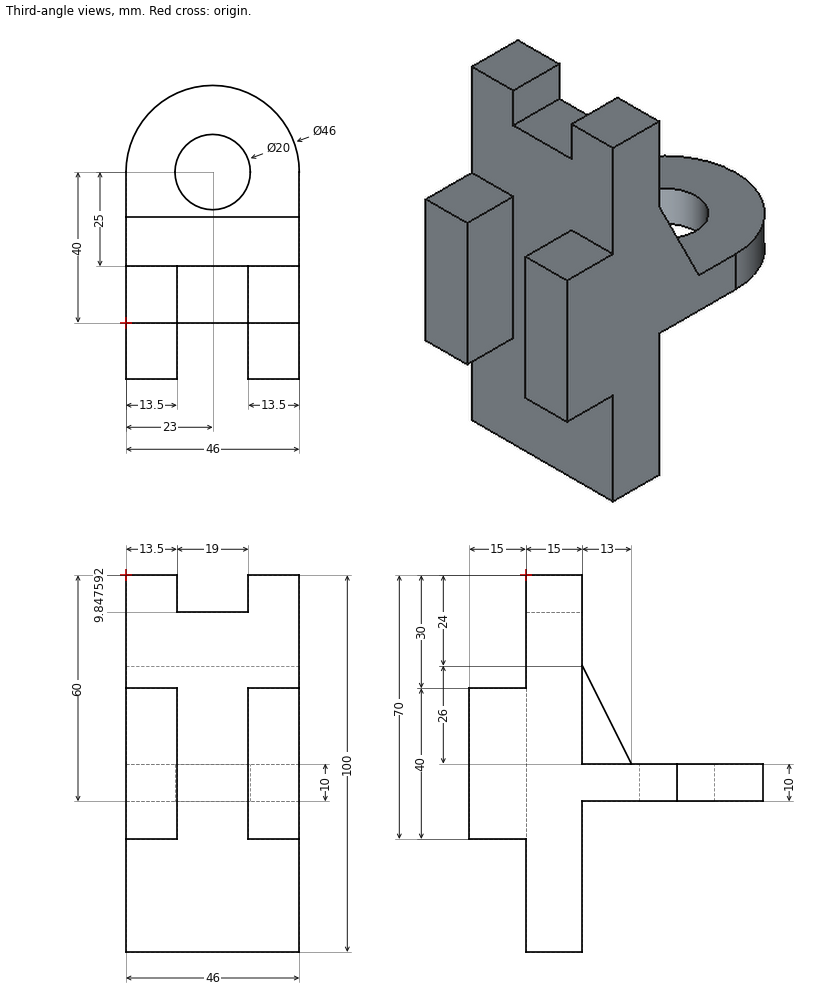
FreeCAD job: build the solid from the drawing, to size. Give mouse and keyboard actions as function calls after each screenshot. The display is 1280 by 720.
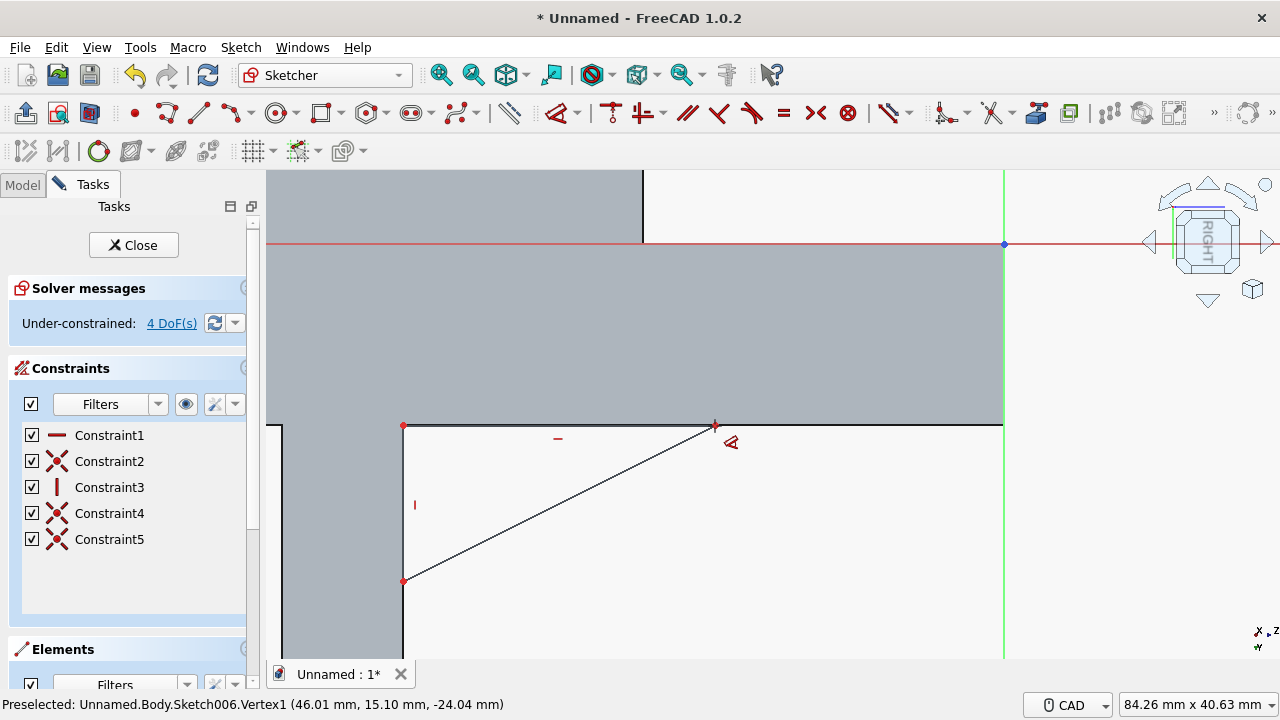
click(621, 426)
click(559, 460)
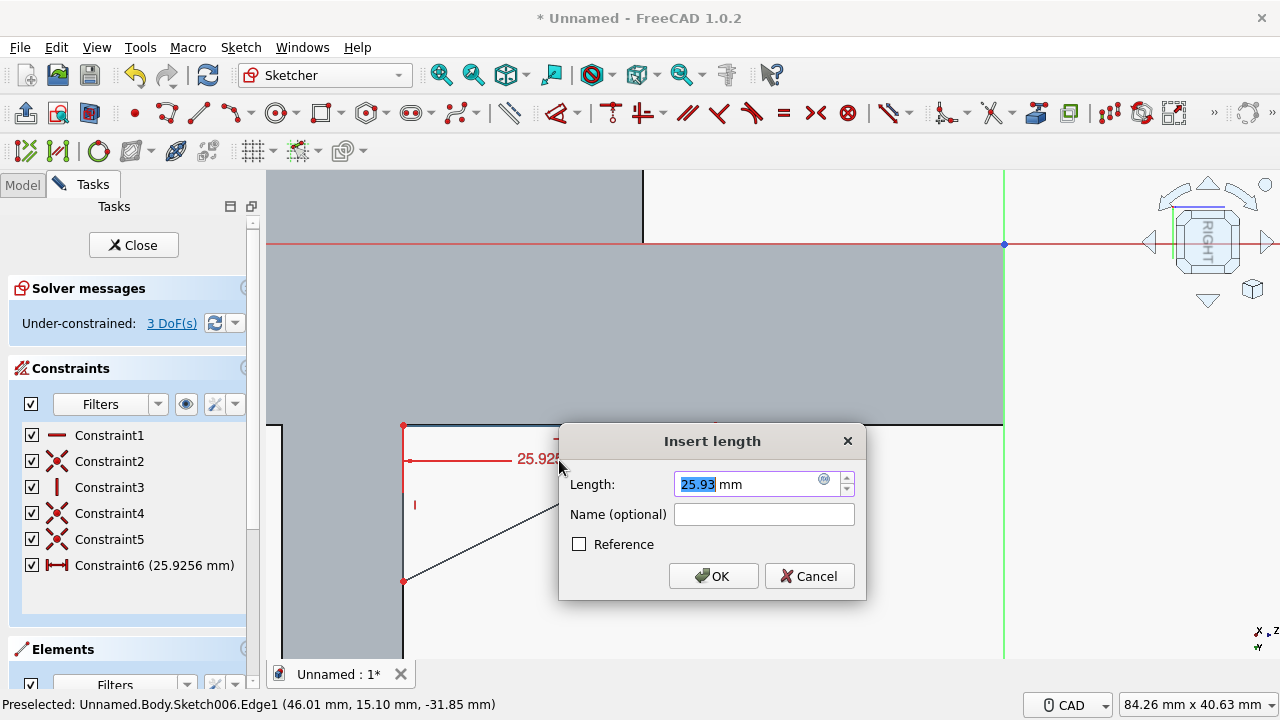
text(26)
key(Return)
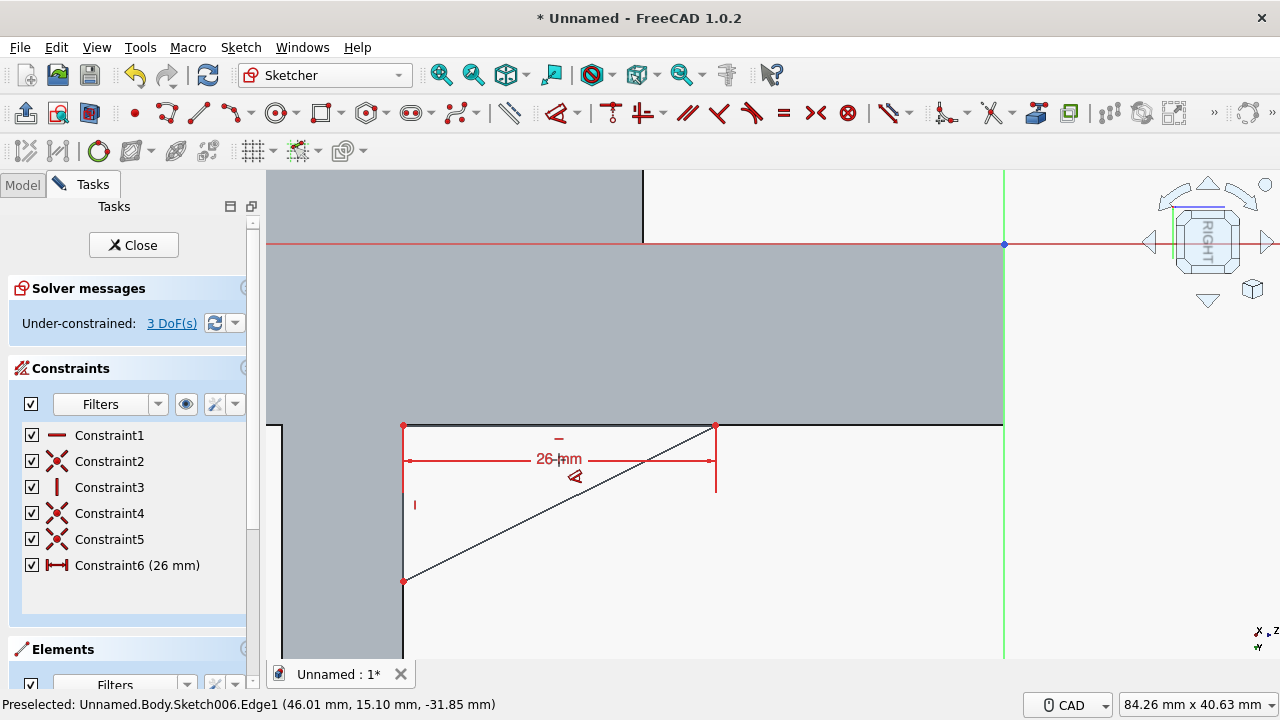
click(403, 473)
click(369, 504)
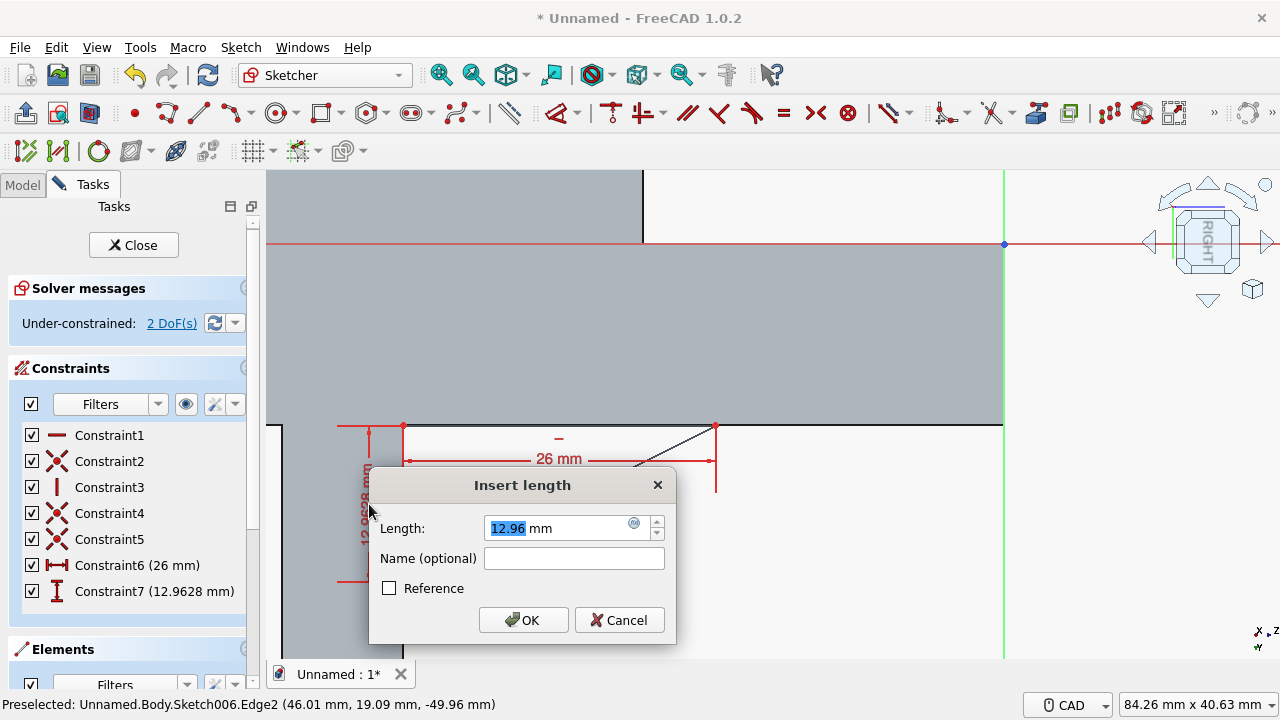
text(13)
key(Return)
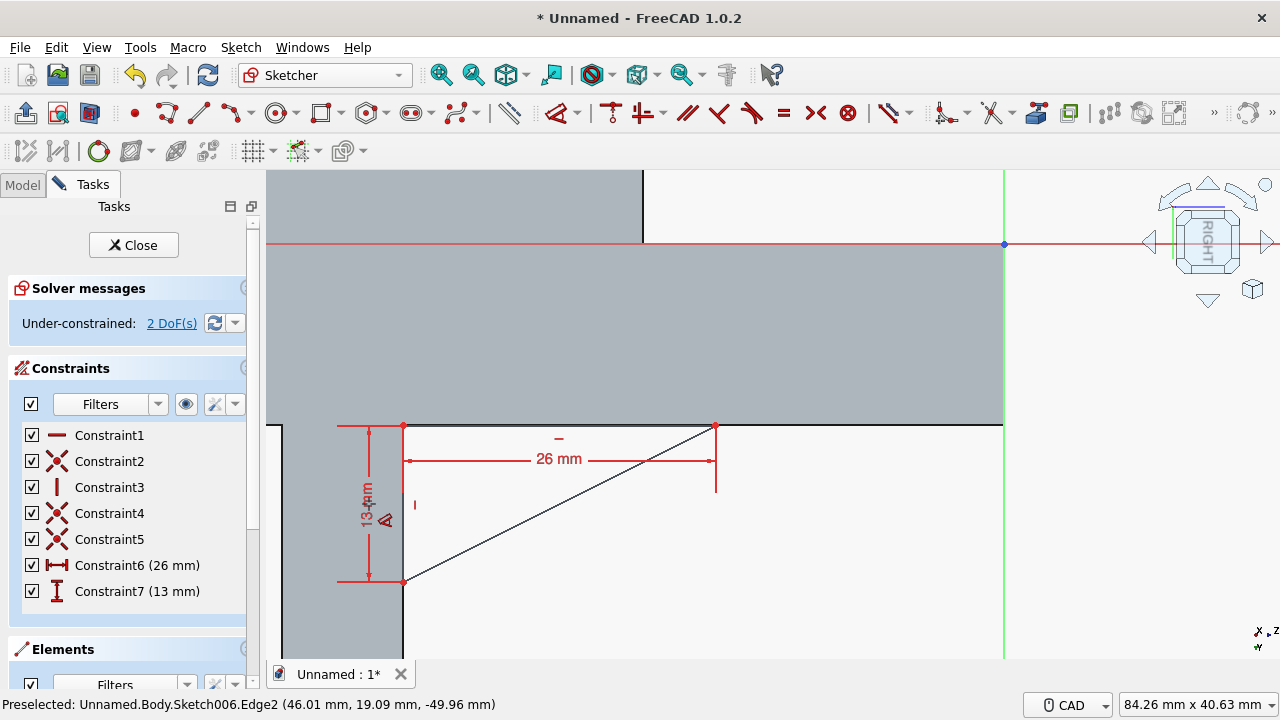
click(716, 426)
click(860, 210)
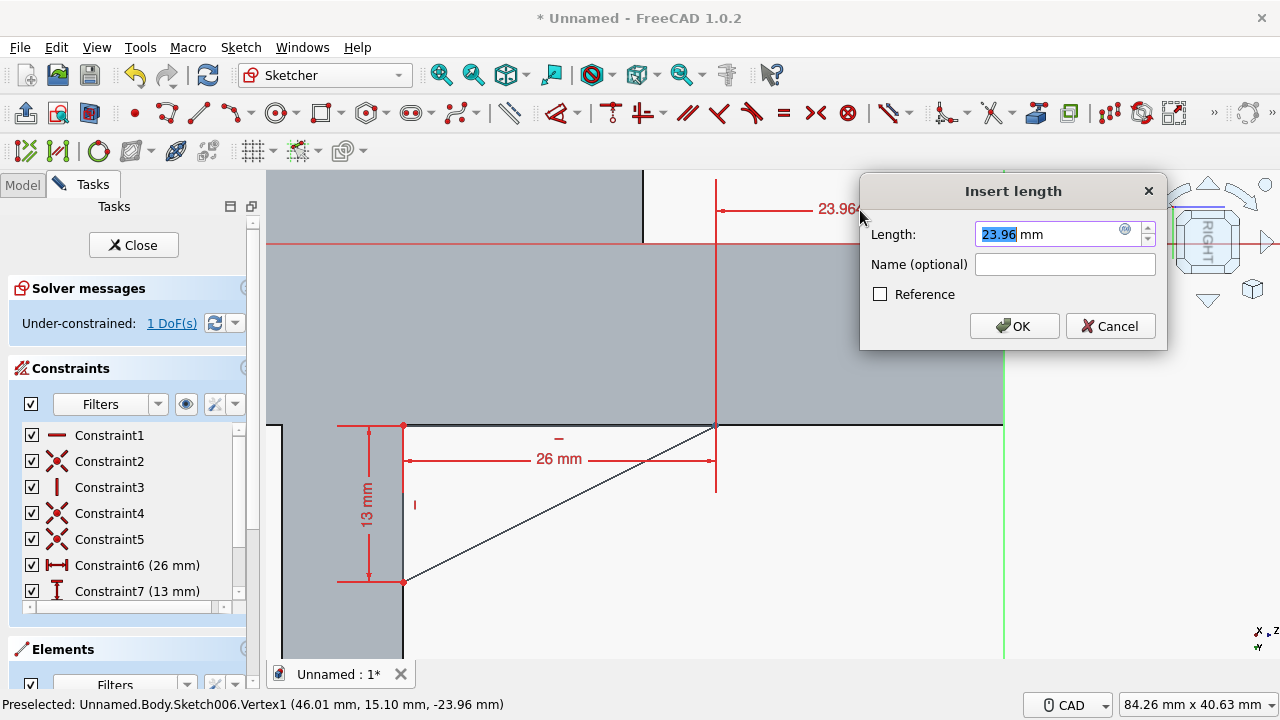
text(24)
key(Return)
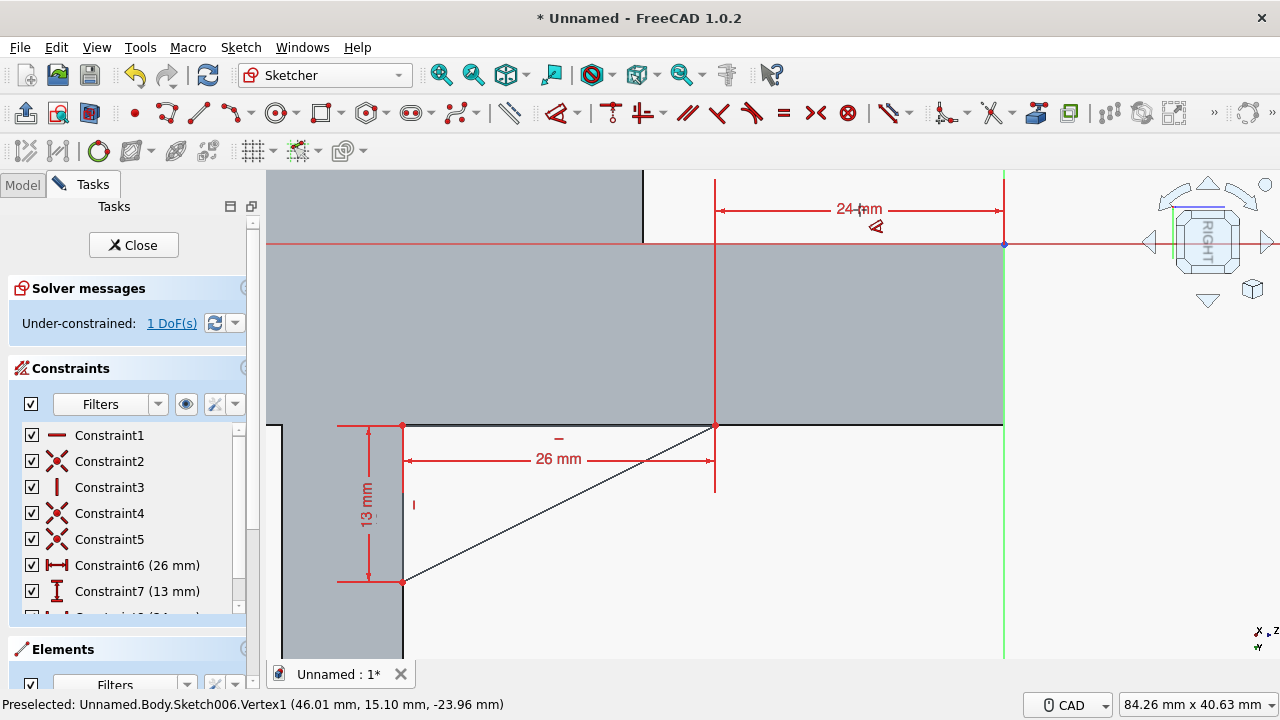
click(715, 426)
click(1038, 335)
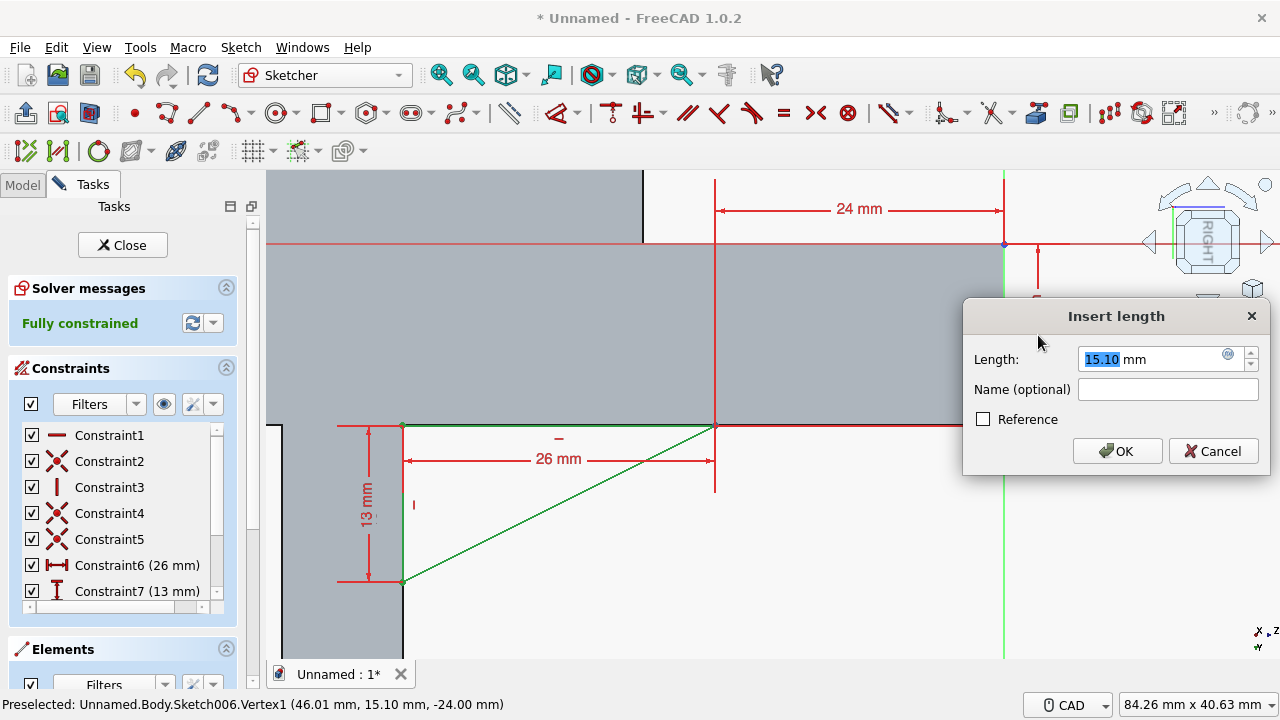
text(15)
key(Return)
key(Escape)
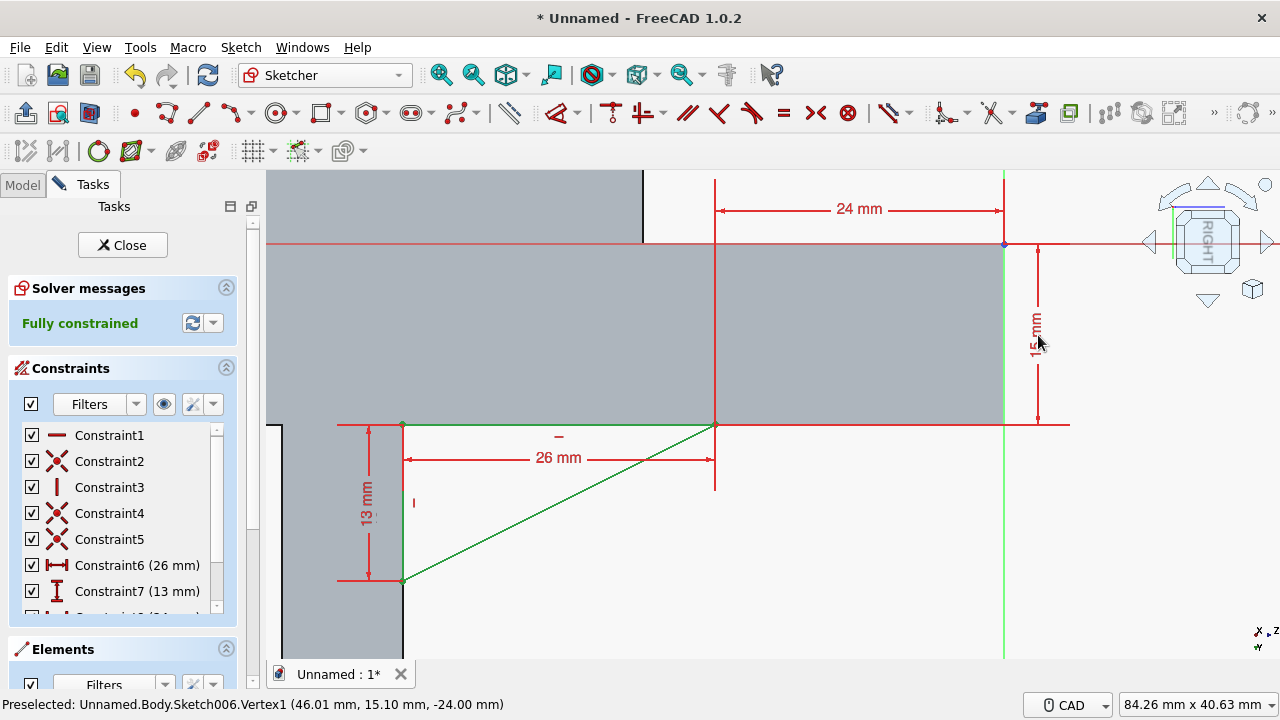
click(123, 245)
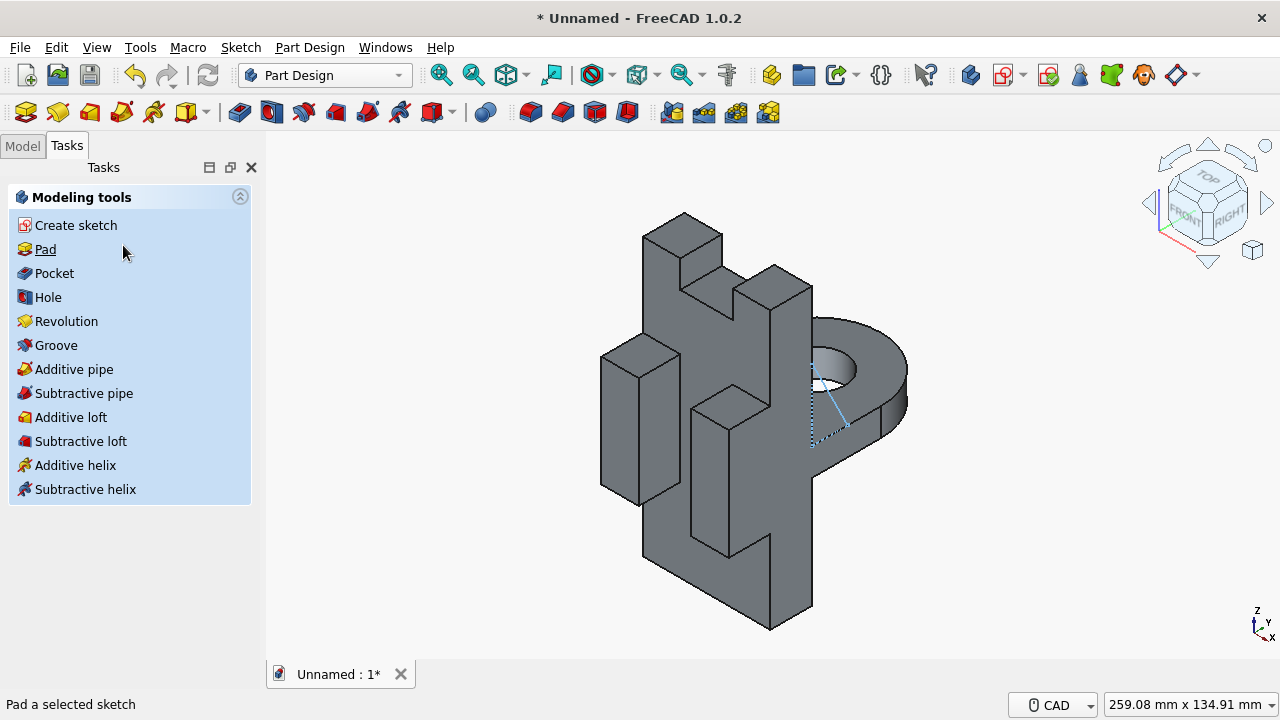
click(26, 112)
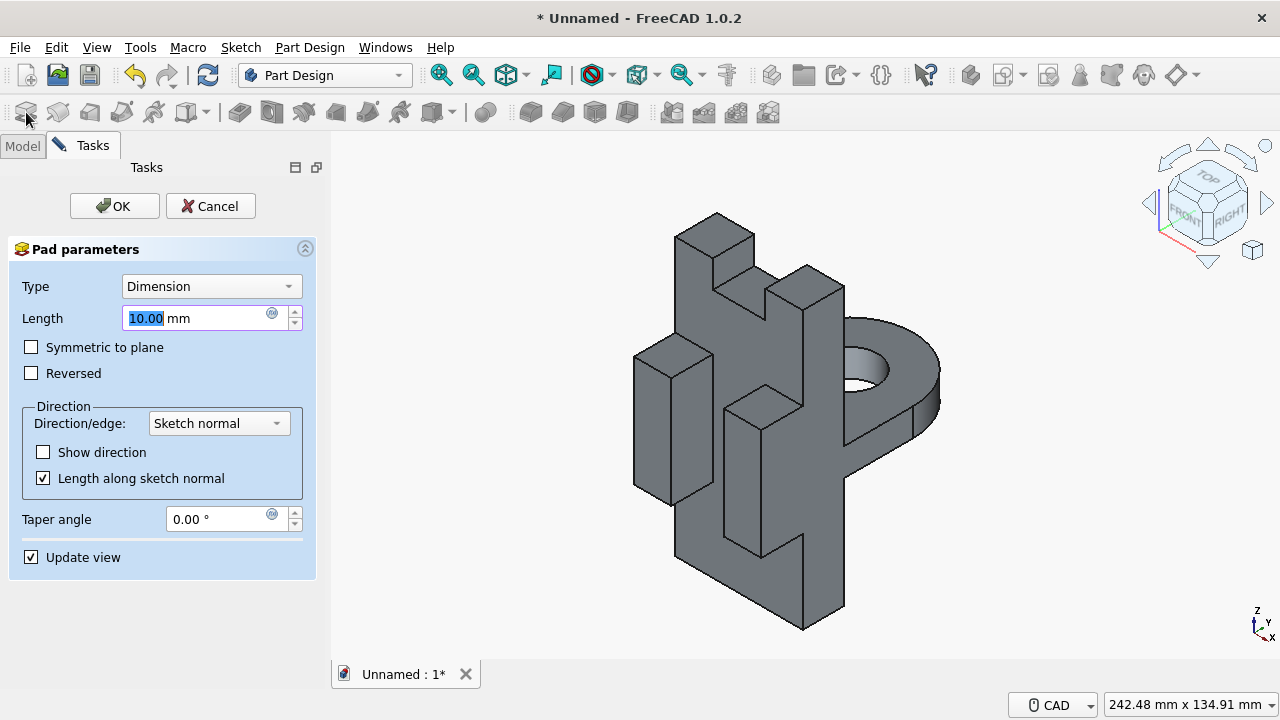
text(46)
key(Tab)